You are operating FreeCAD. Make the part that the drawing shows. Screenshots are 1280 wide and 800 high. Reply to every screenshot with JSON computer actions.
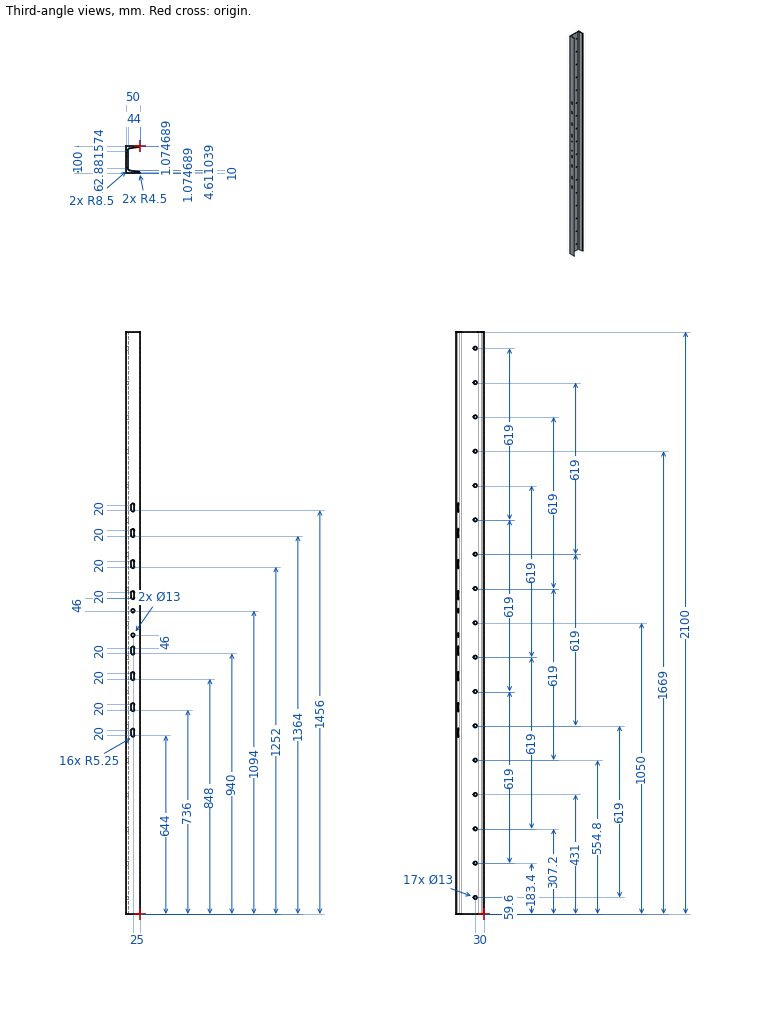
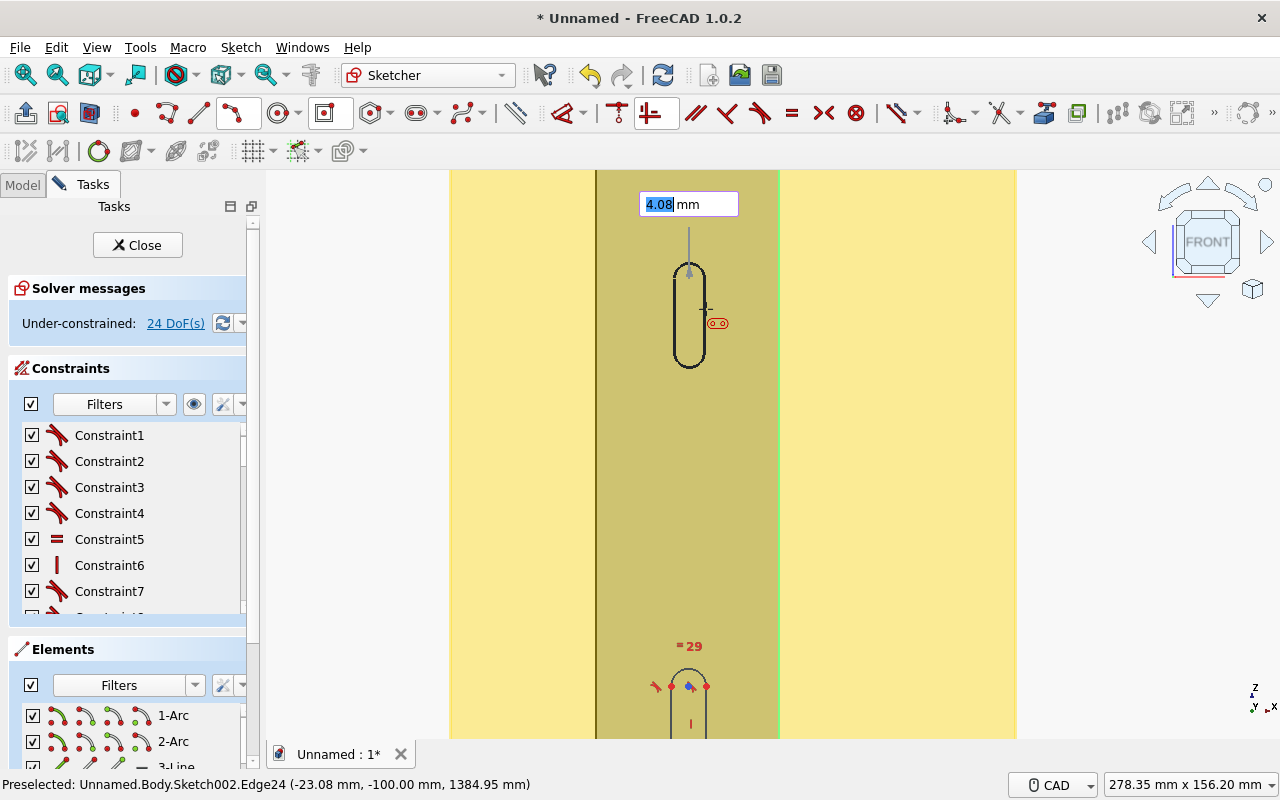
{"action": "left_click", "coordinate": [707, 309]}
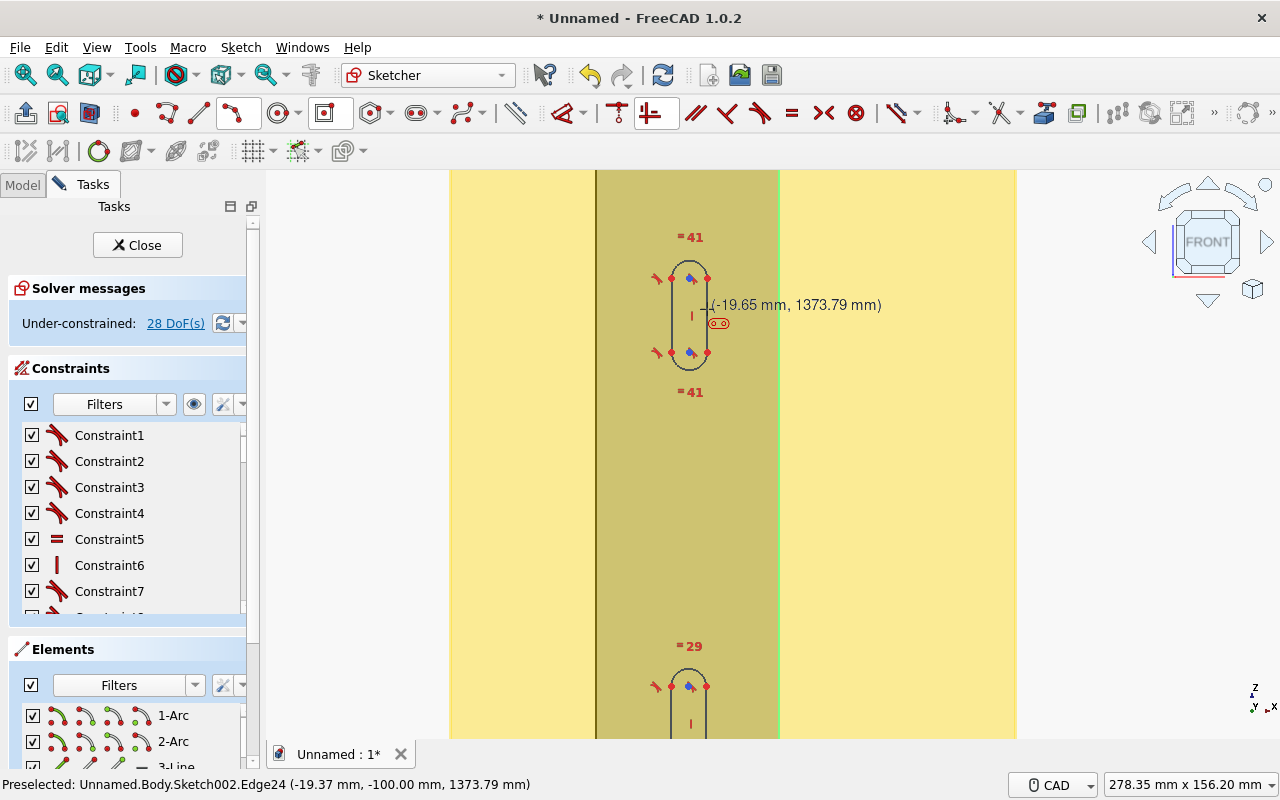
{"action": "scroll", "coordinate": [703, 315], "scroll_direction": "down", "scroll_amount": 14}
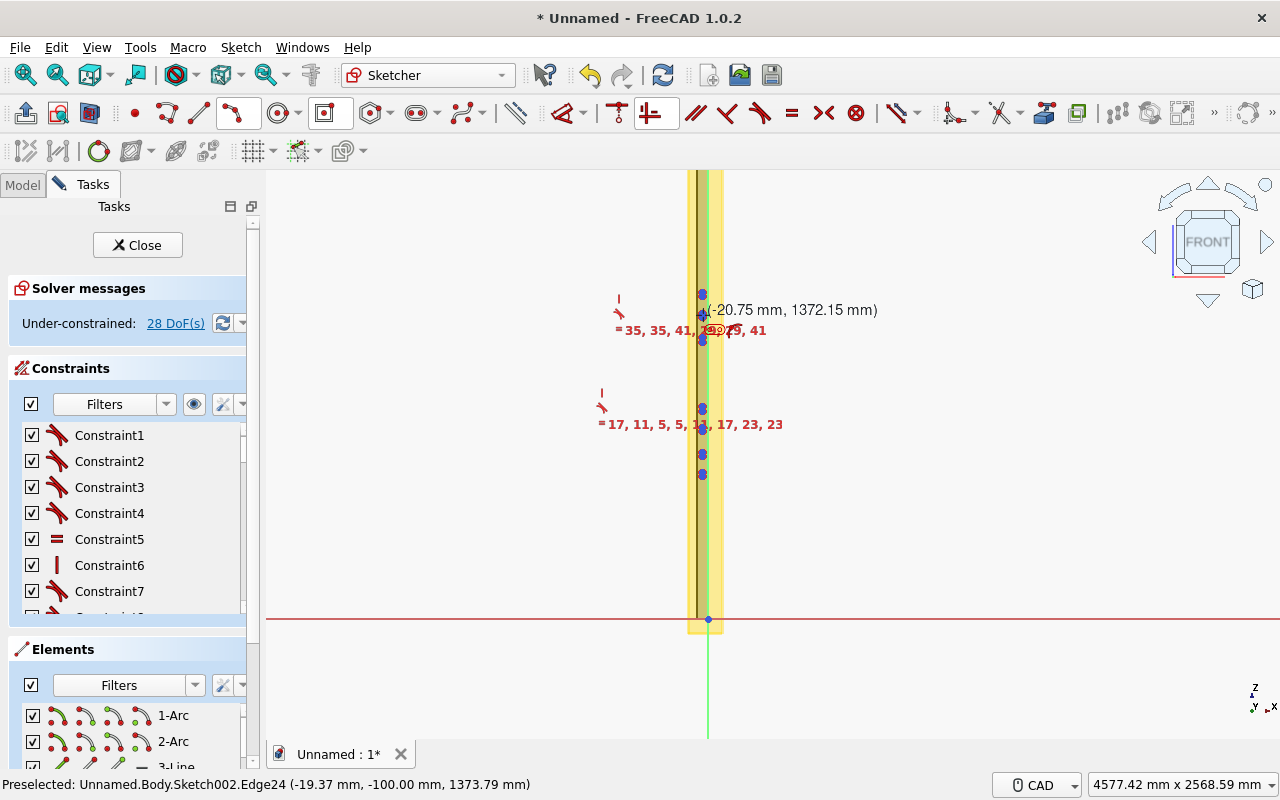
{"action": "scroll", "coordinate": [702, 367], "scroll_direction": "up", "scroll_amount": 15}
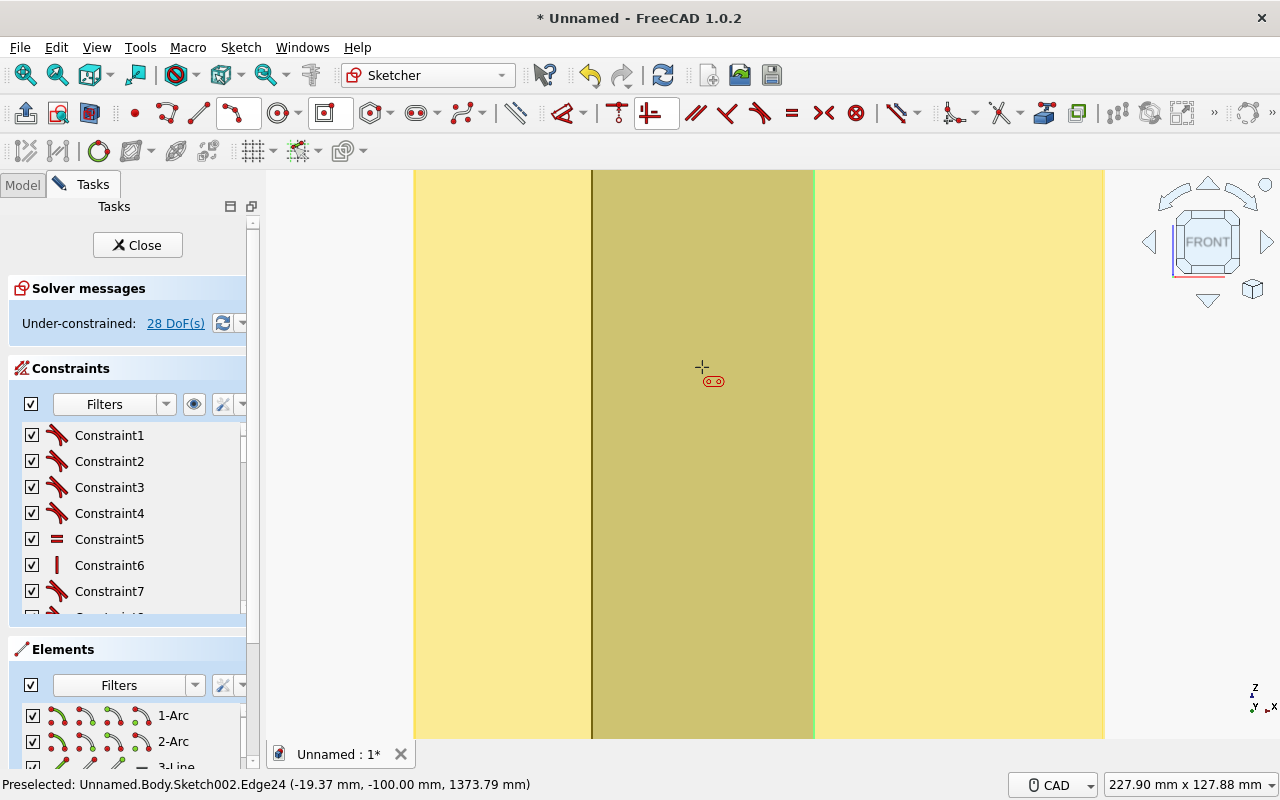
{"action": "scroll", "coordinate": [702, 367], "scroll_direction": "down", "scroll_amount": 15}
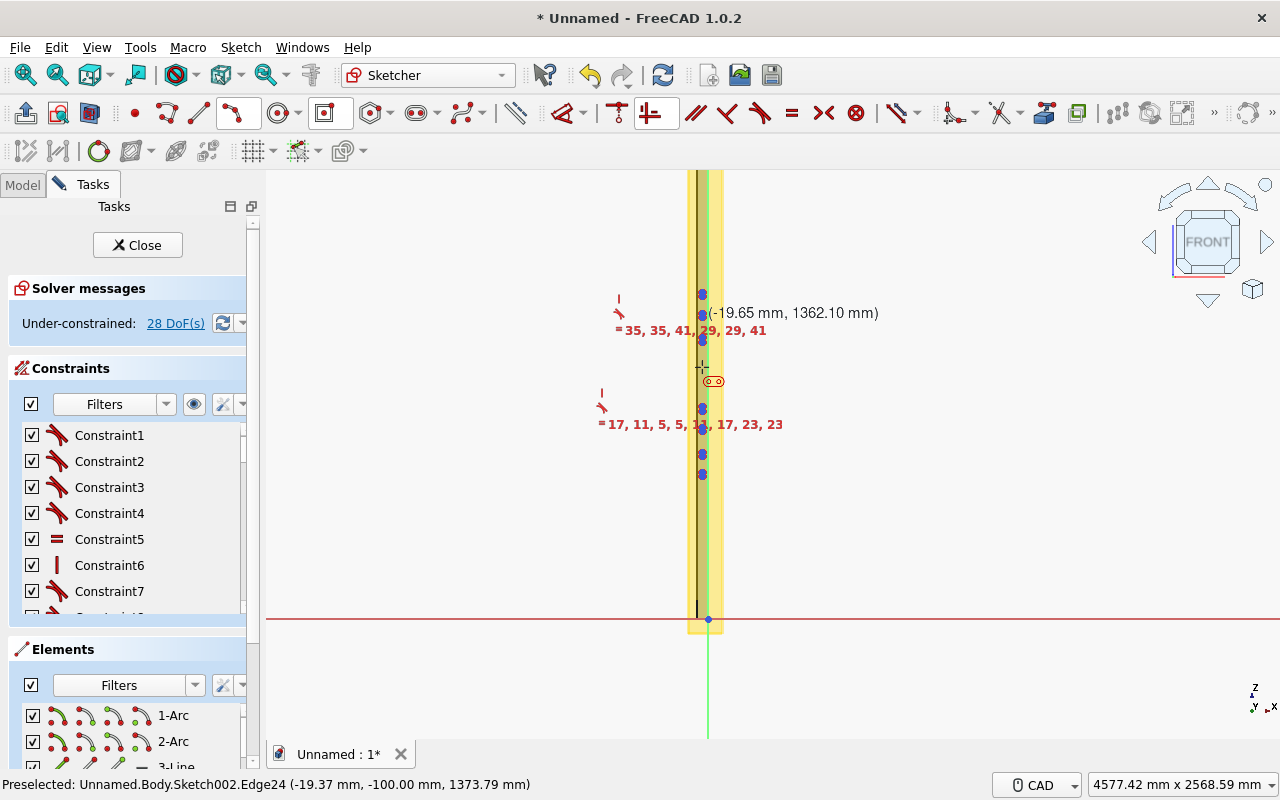
{"action": "scroll", "coordinate": [702, 367], "scroll_direction": "up", "scroll_amount": 6}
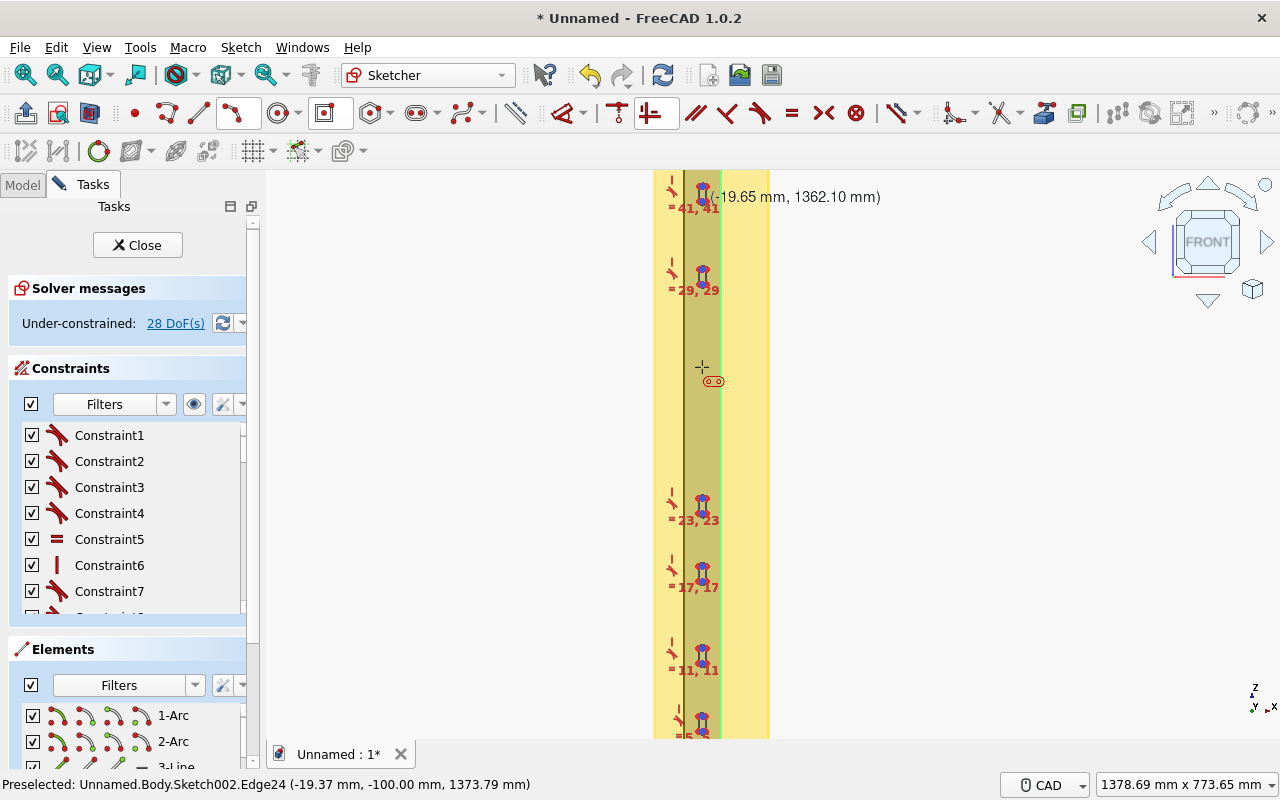
{"action": "left_click", "coordinate": [703, 365]}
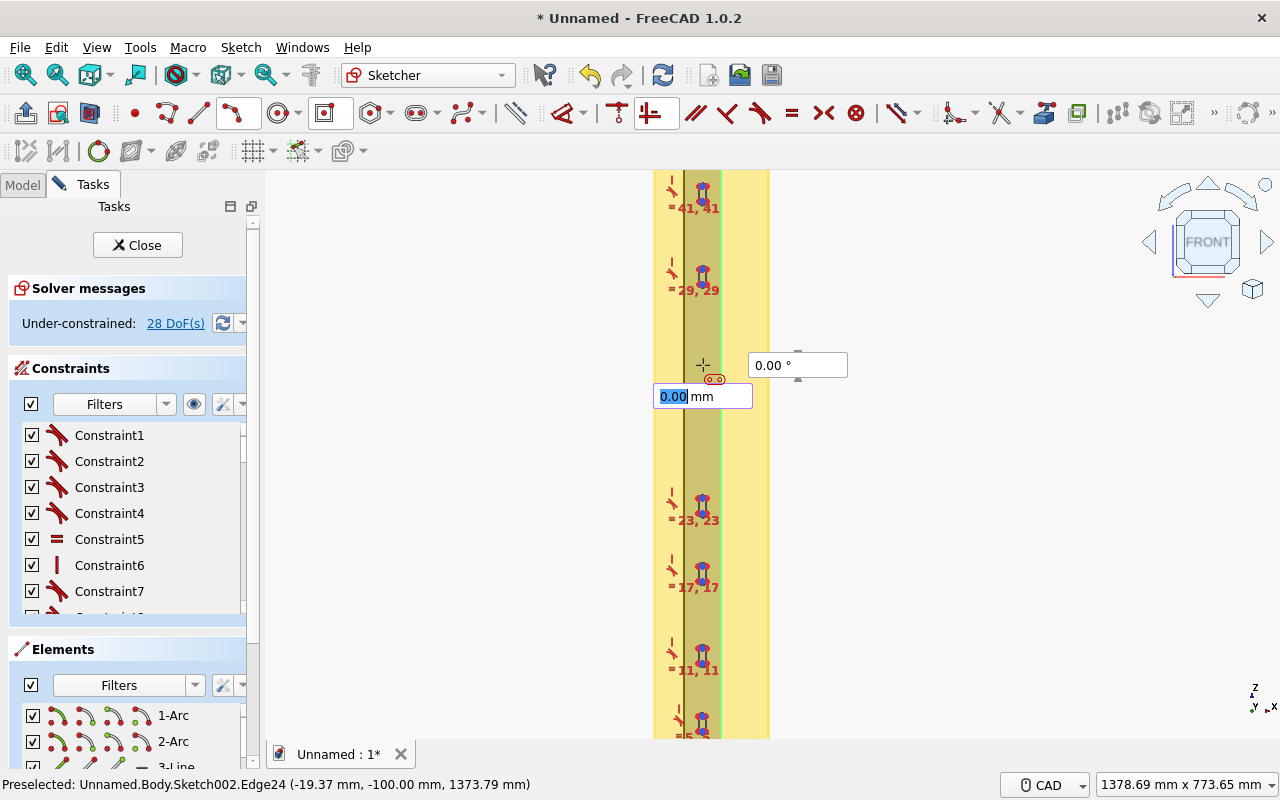
{"action": "left_click", "coordinate": [703, 351]}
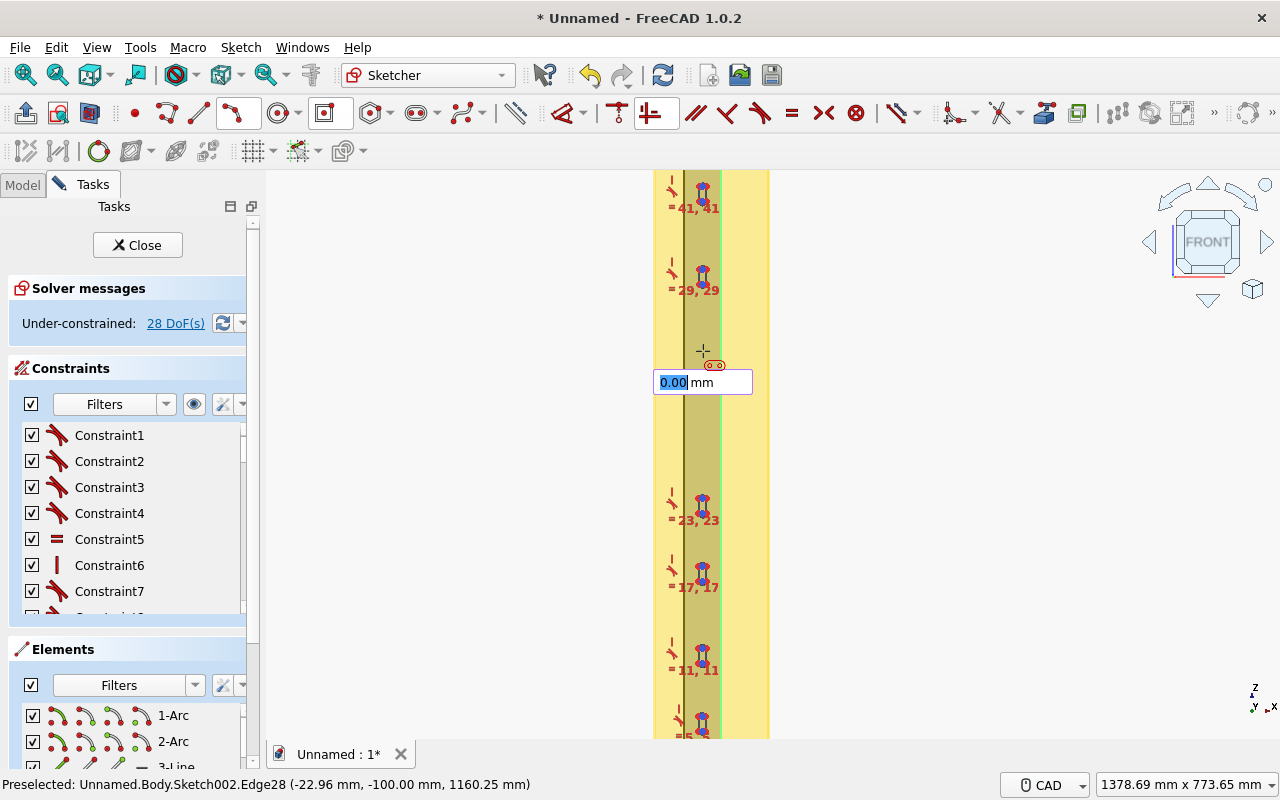
{"action": "scroll", "coordinate": [706, 358], "scroll_direction": "up", "scroll_amount": 8}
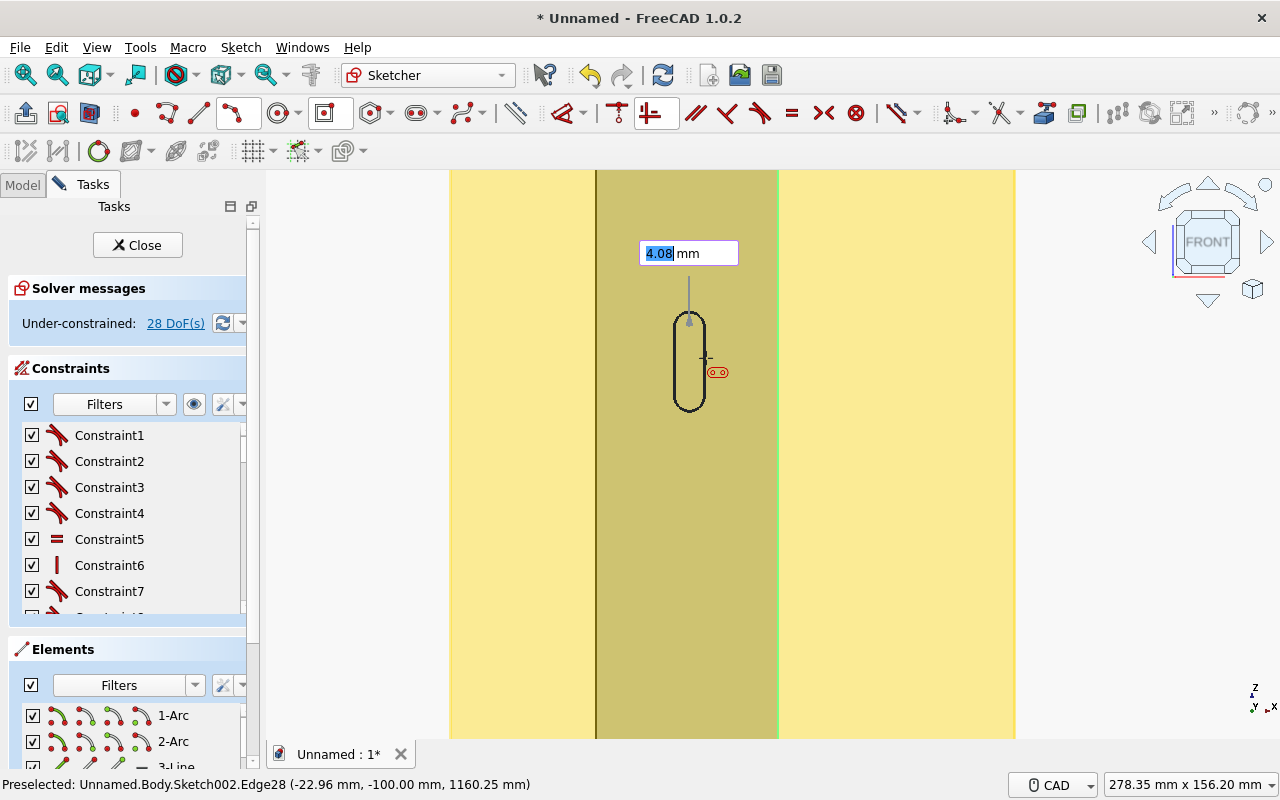
{"action": "left_click", "coordinate": [706, 356]}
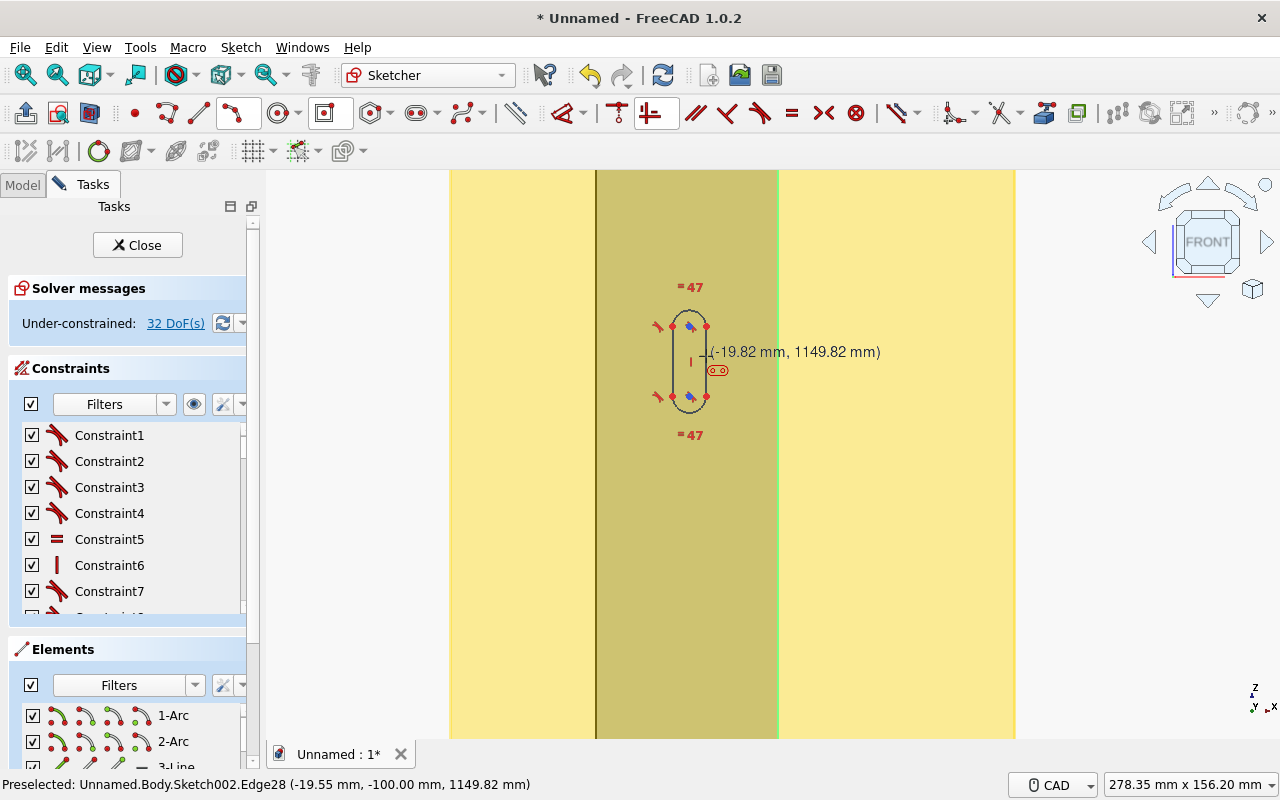
{"action": "left_click", "coordinate": [278, 114]}